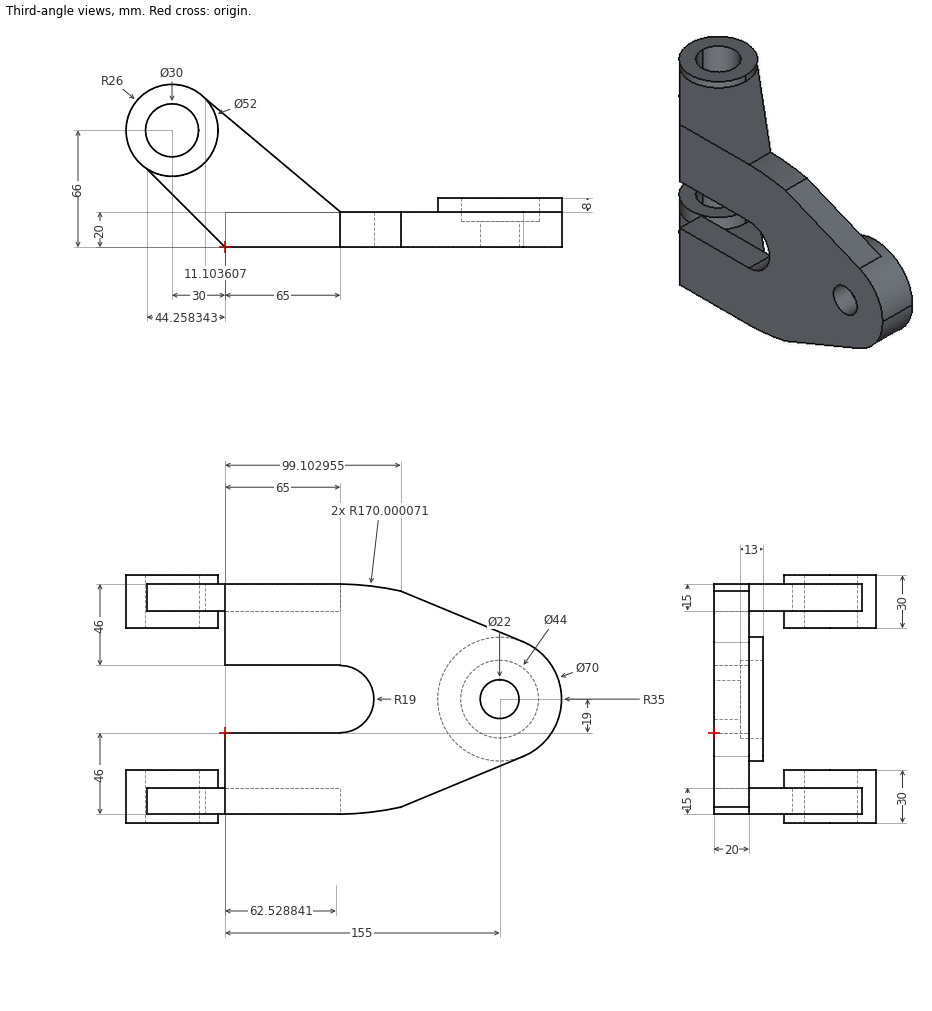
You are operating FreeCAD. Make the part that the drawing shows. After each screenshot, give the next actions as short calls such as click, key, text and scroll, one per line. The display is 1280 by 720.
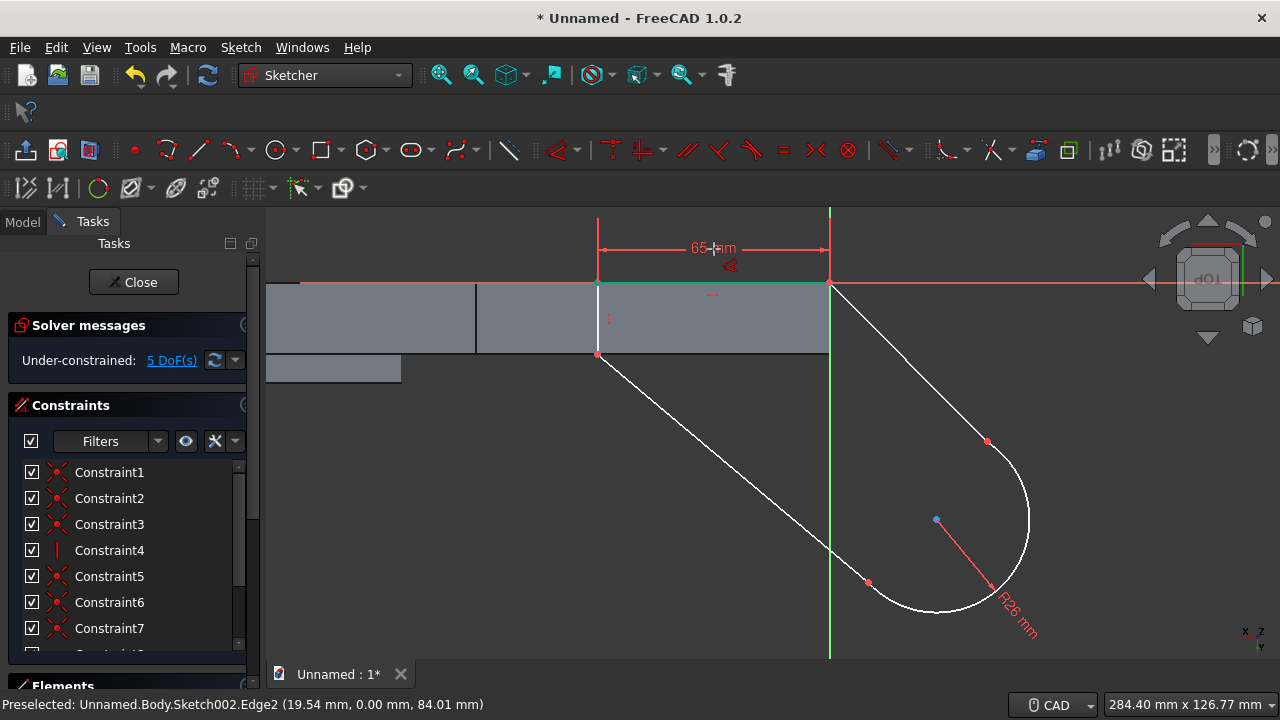
click(598, 304)
click(564, 319)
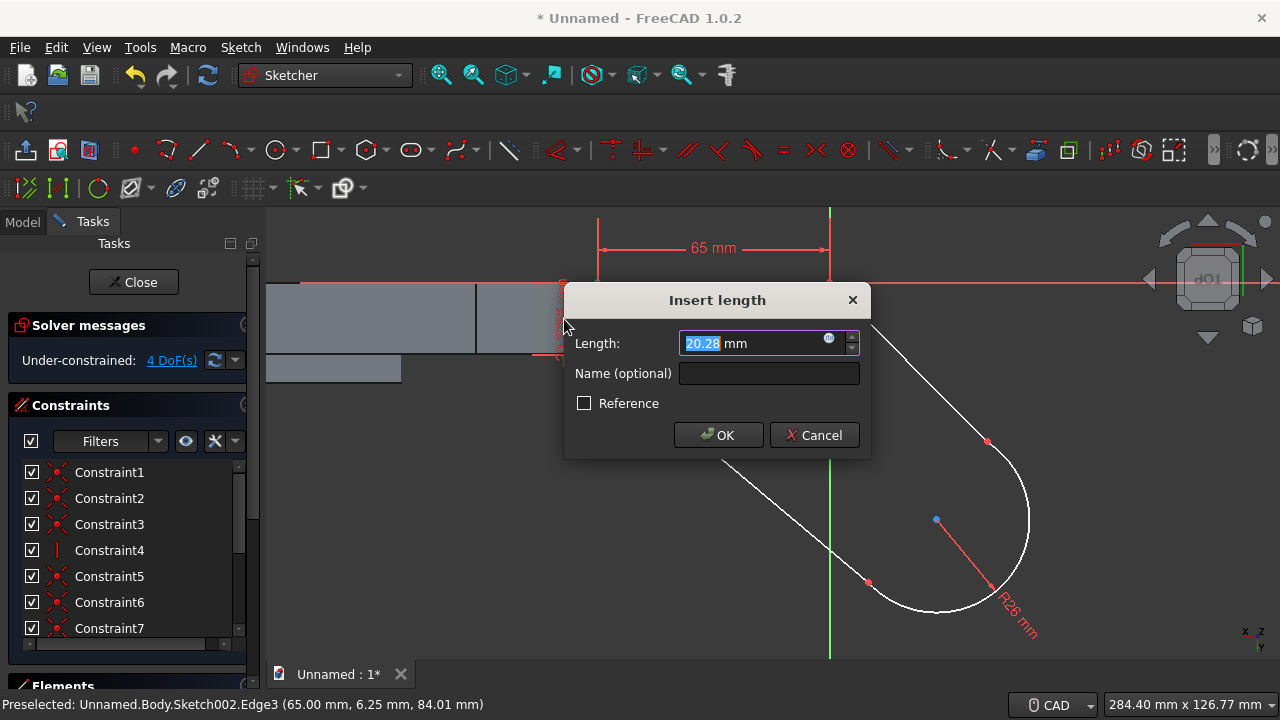
text(20)
key(Return)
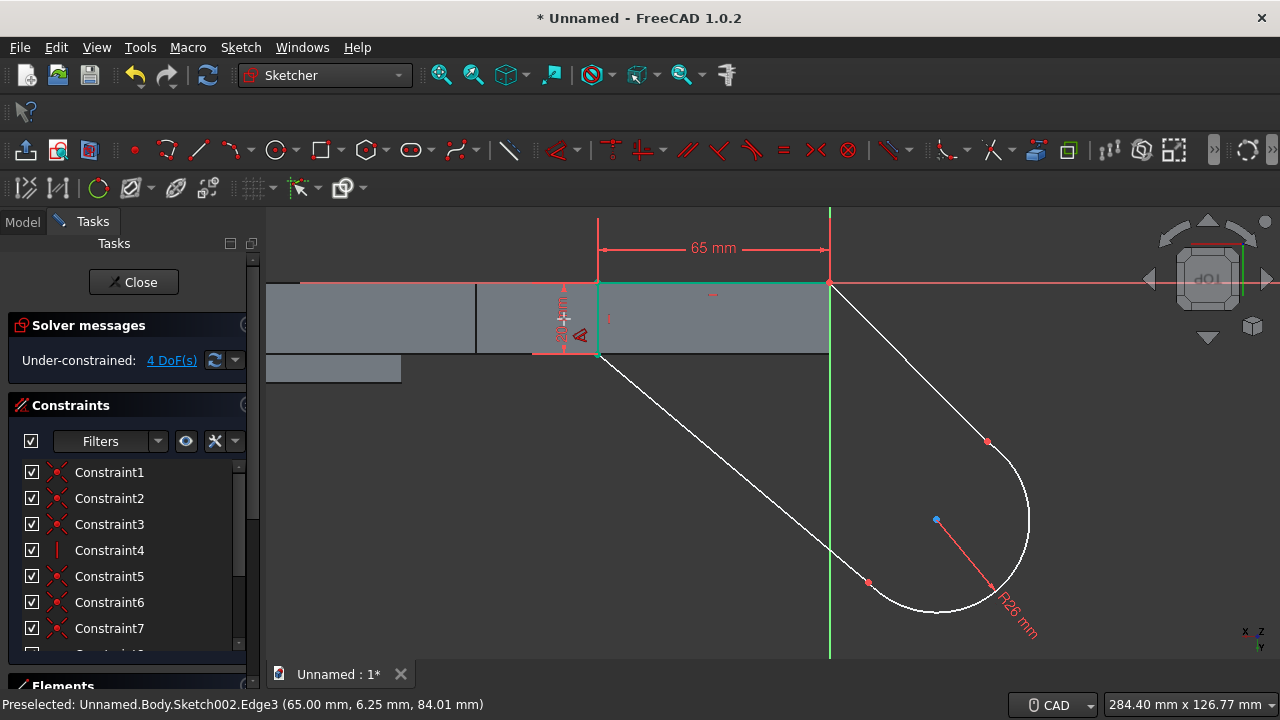
click(937, 520)
click(883, 249)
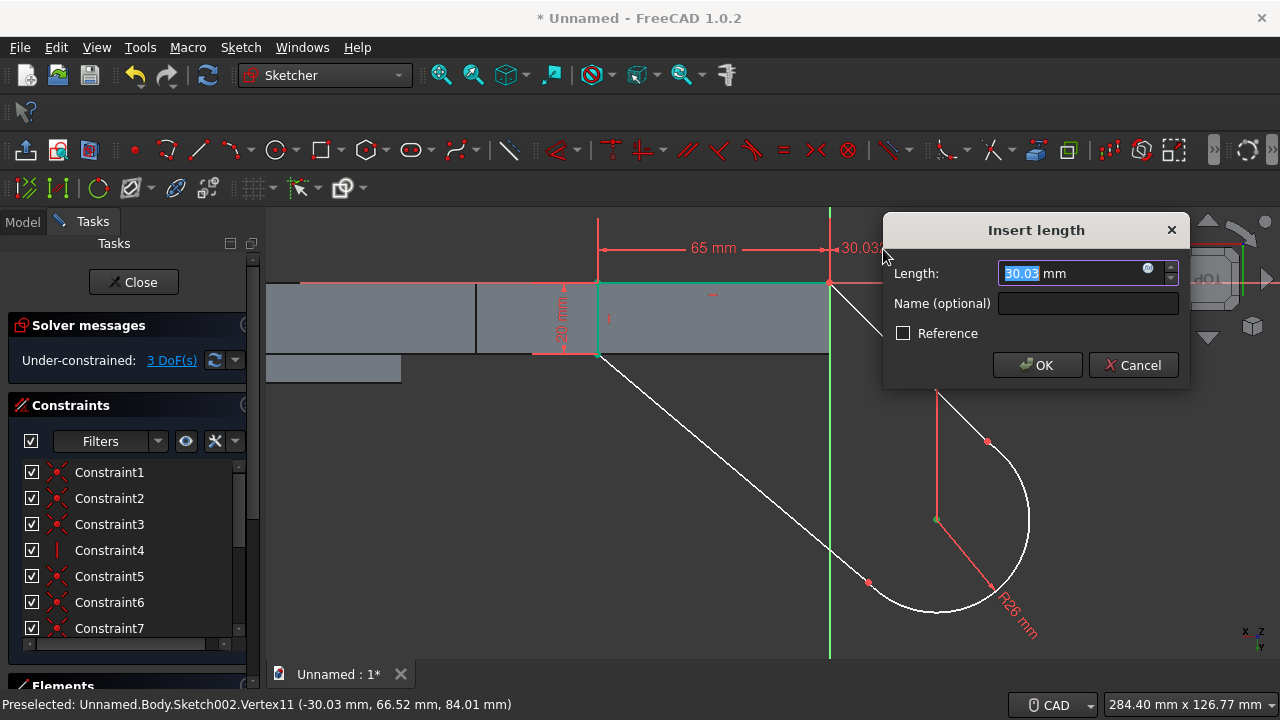
text(30)
key(Return)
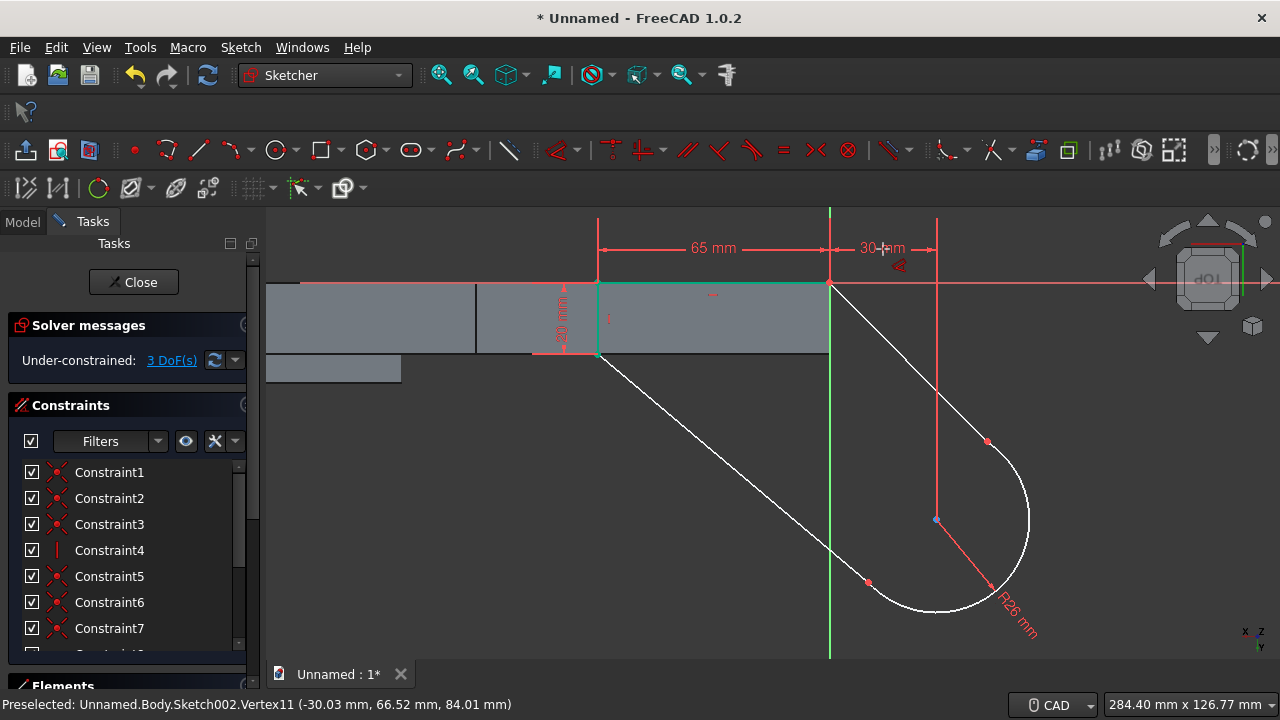
click(937, 520)
click(971, 401)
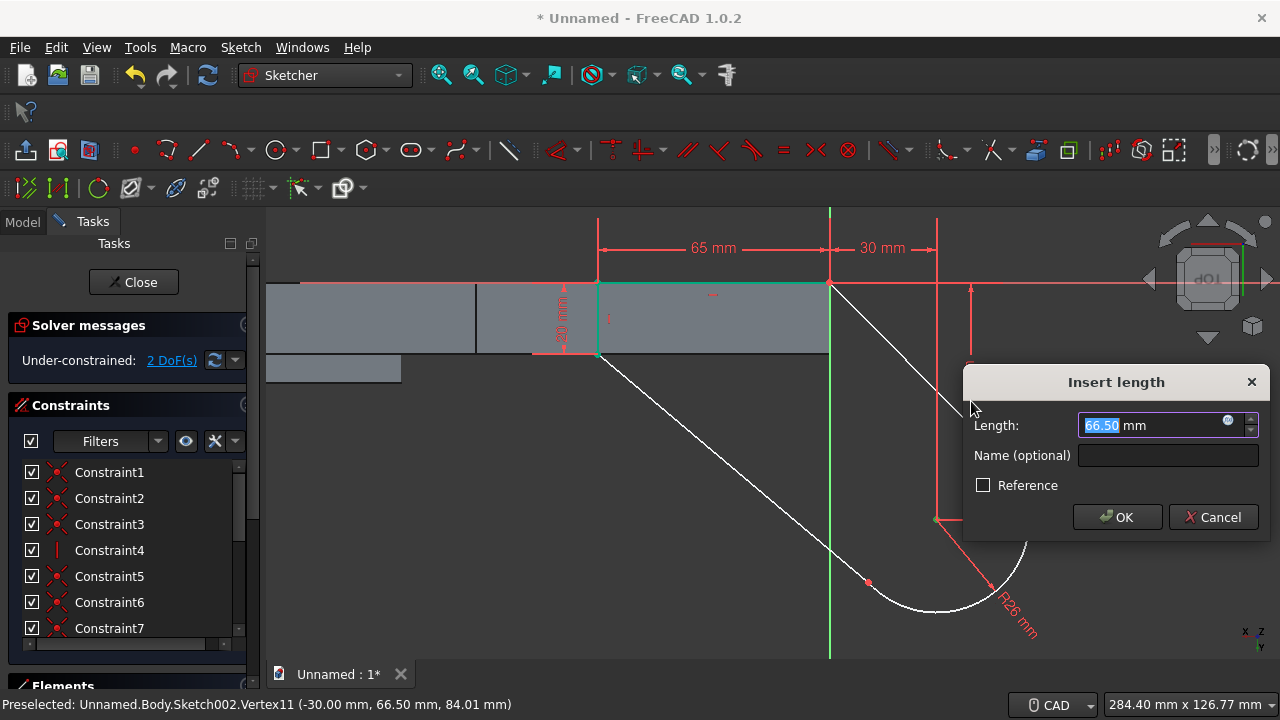
text(66)
key(Return)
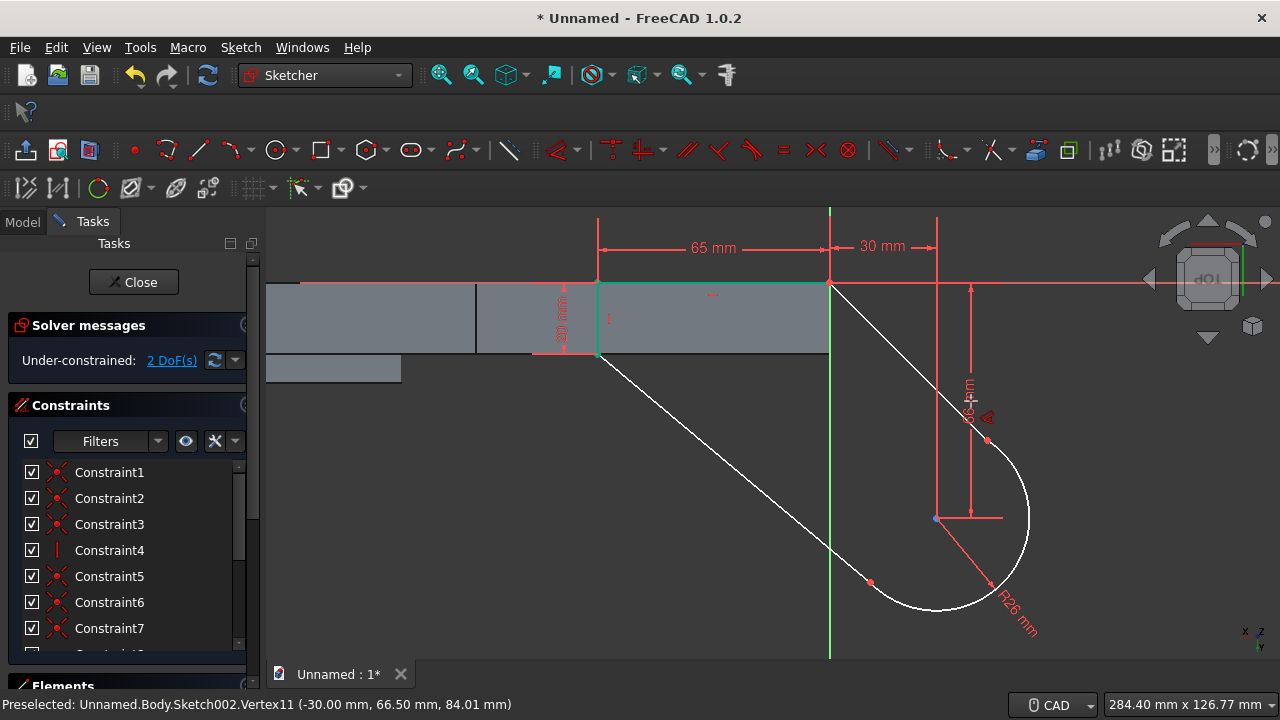
click(987, 440)
click(963, 249)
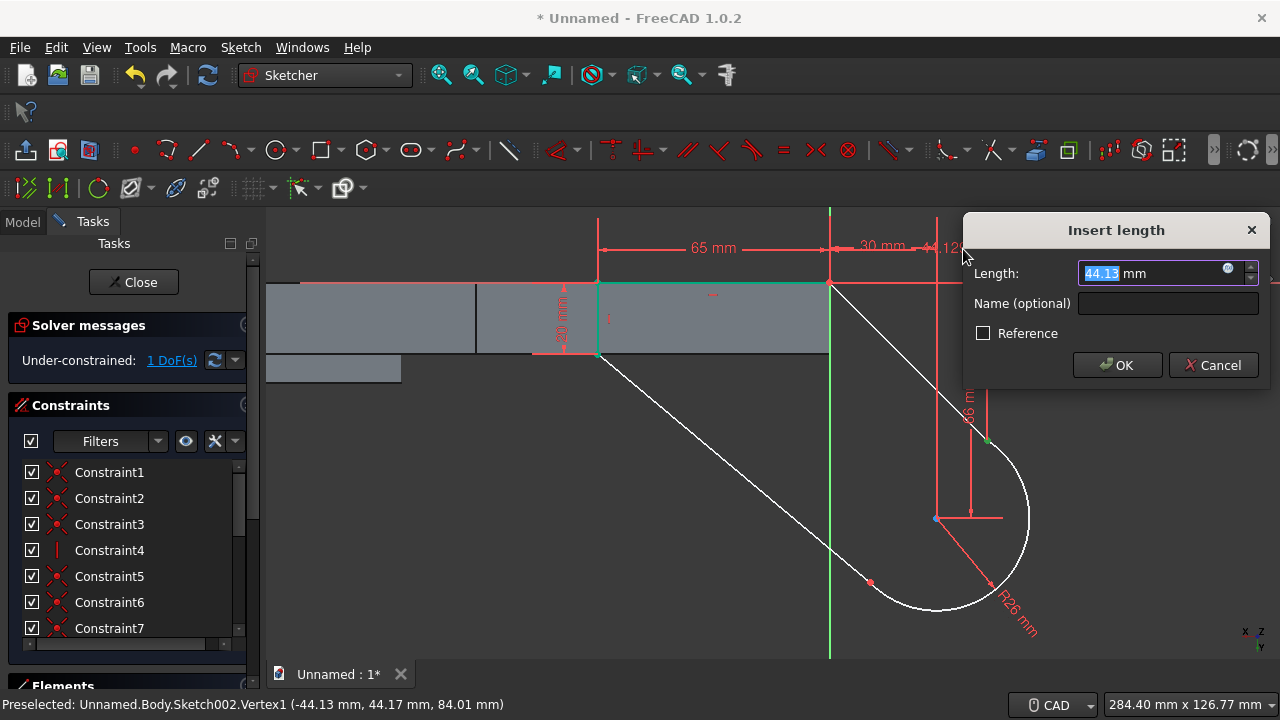
text(44.258343)
key(Return)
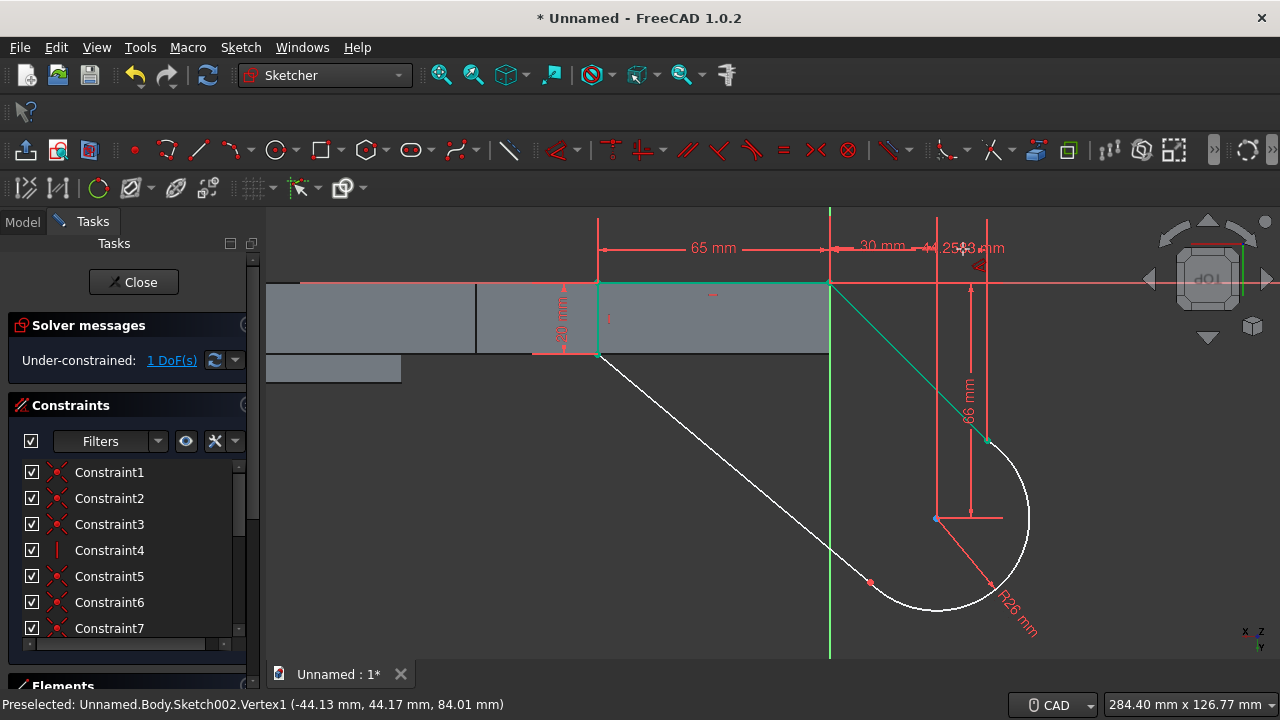
click(871, 583)
click(850, 617)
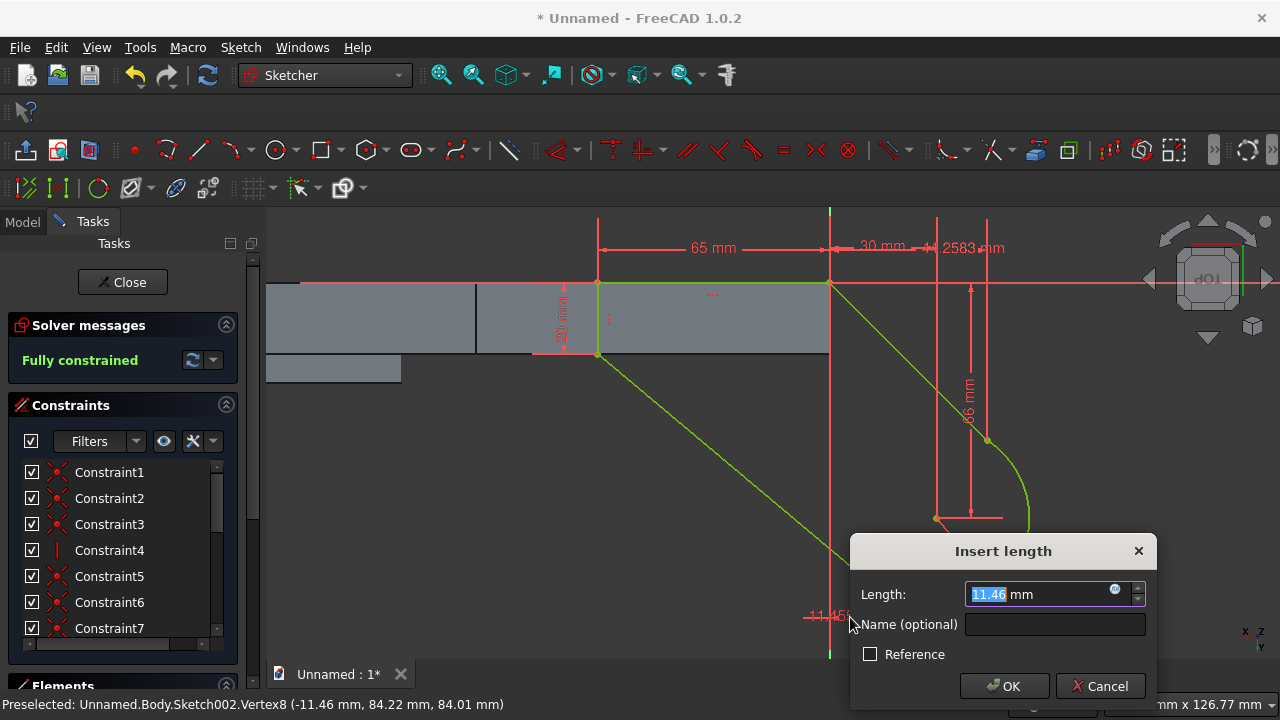
text(11.103607)
key(Return)
key(Escape)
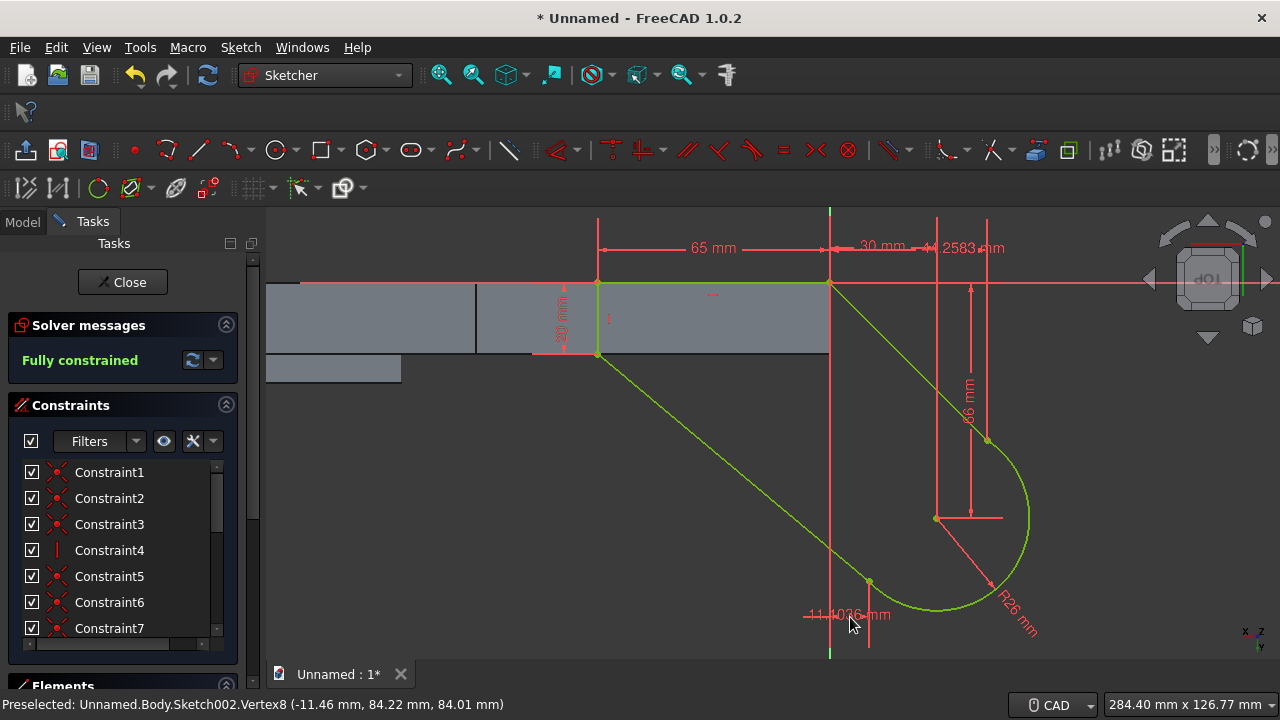
click(123, 282)